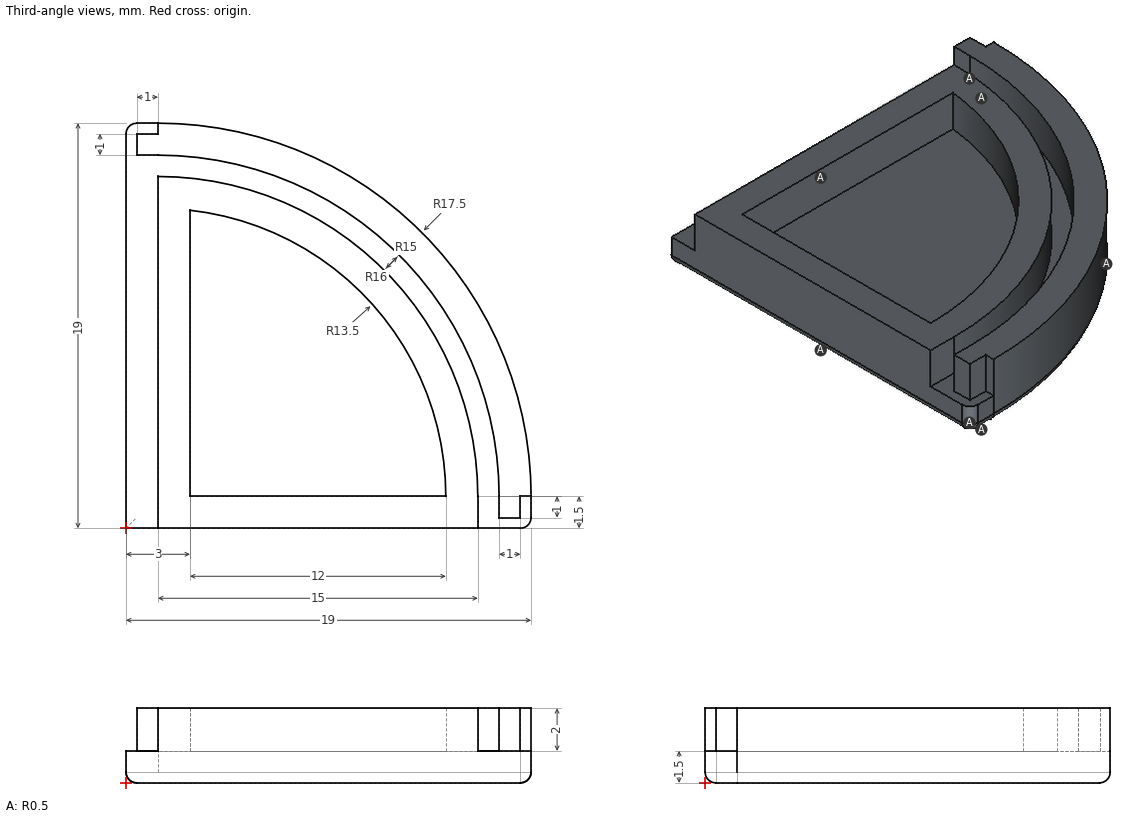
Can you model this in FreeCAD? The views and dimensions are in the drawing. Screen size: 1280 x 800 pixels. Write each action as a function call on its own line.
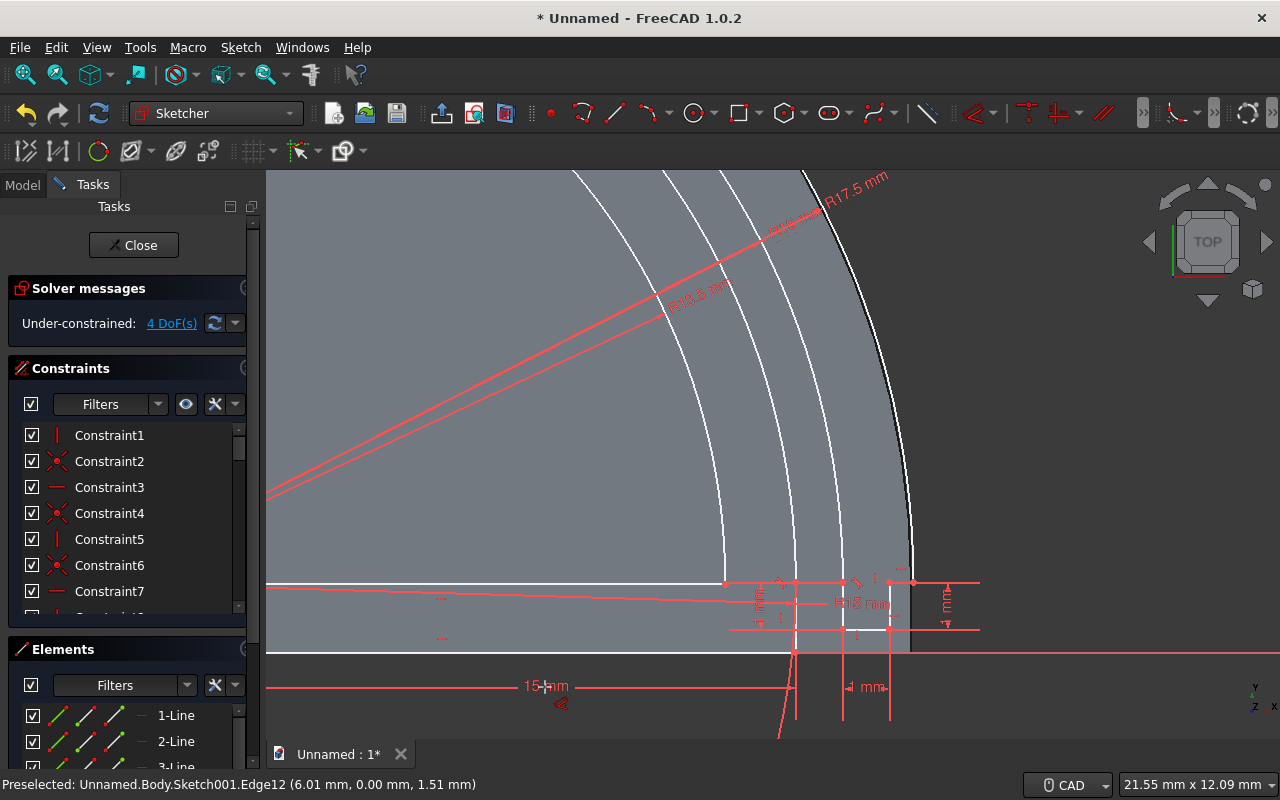
click(555, 584)
click(510, 618)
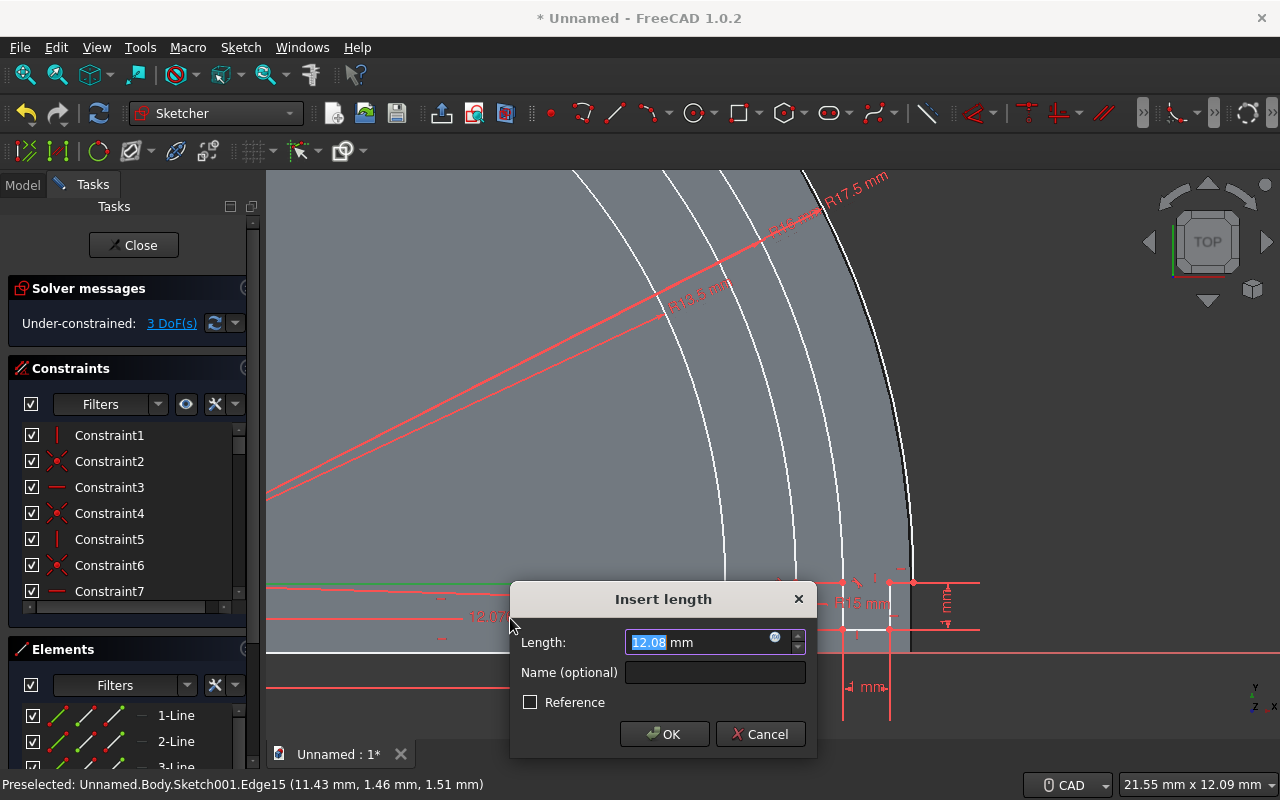
text(12)
key(Return)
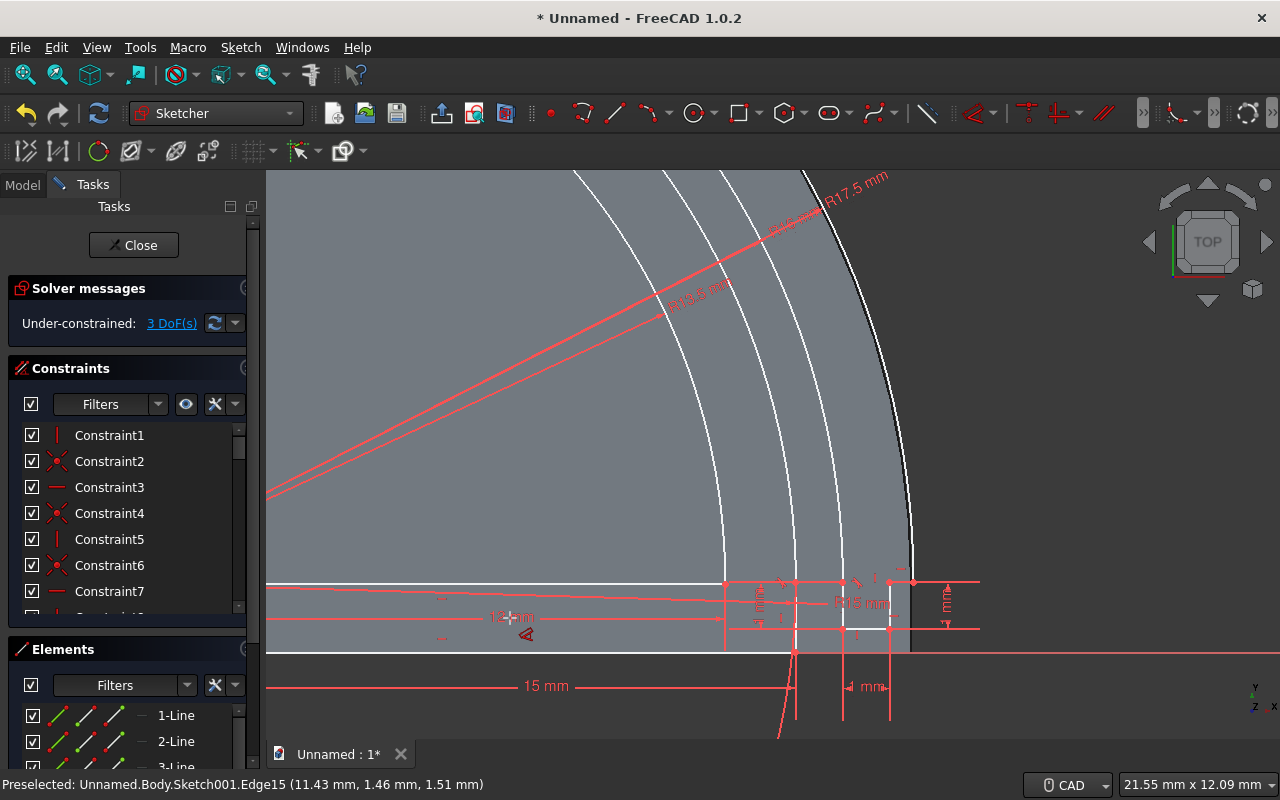
scroll(844, 599, down, 5)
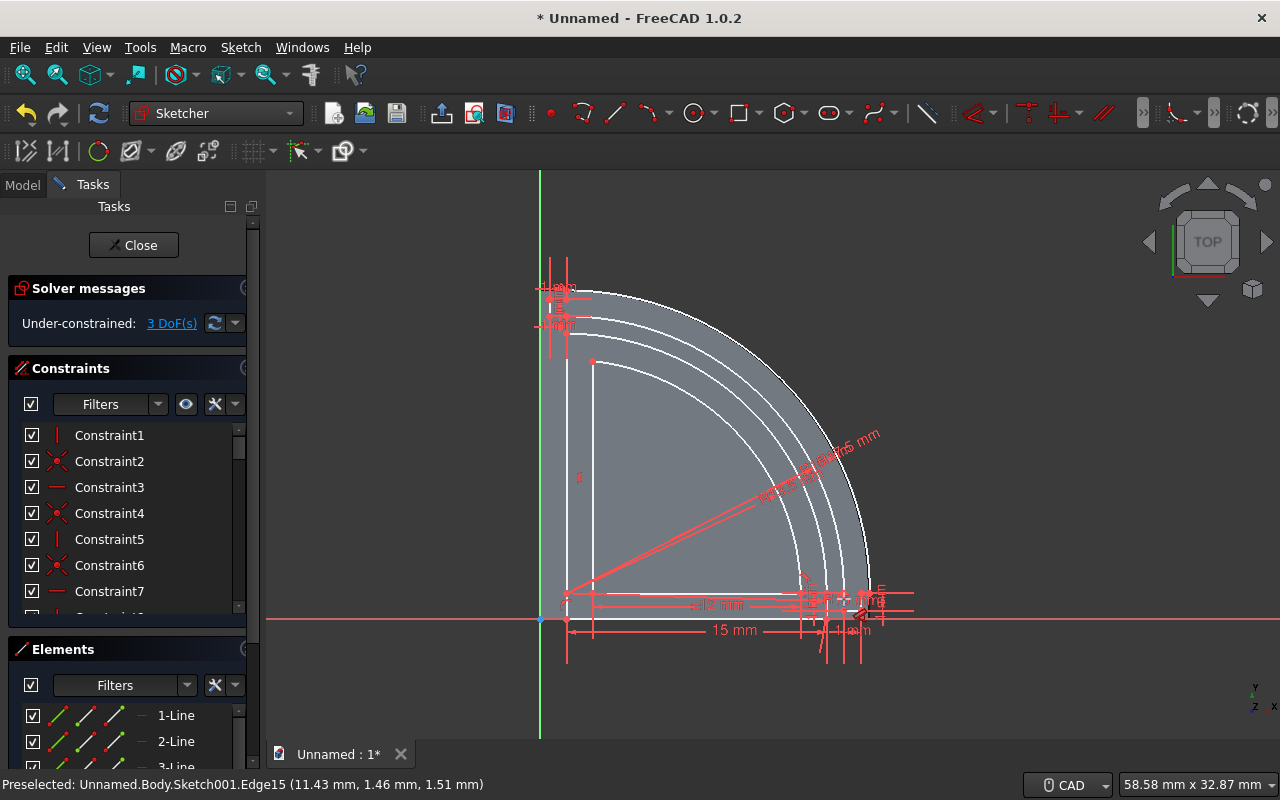
click(593, 594)
click(567, 653)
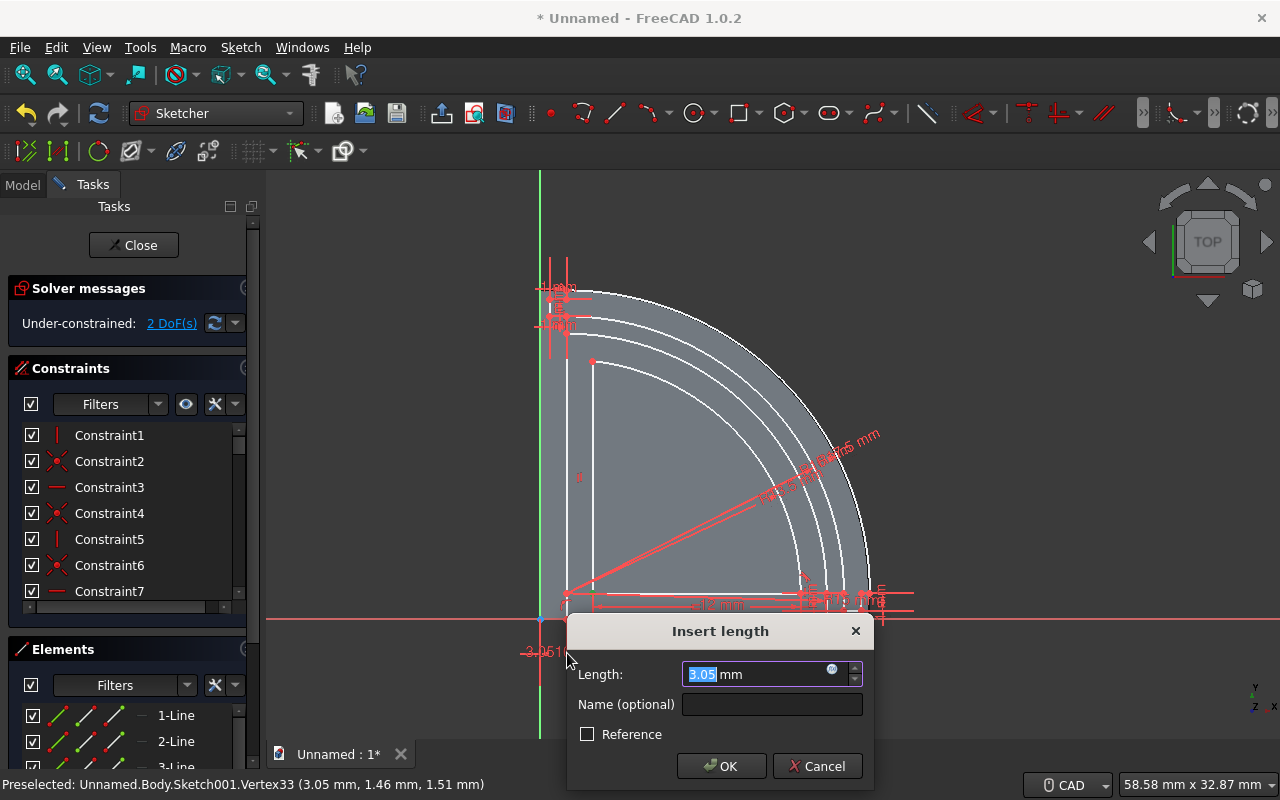
text(3)
key(Return)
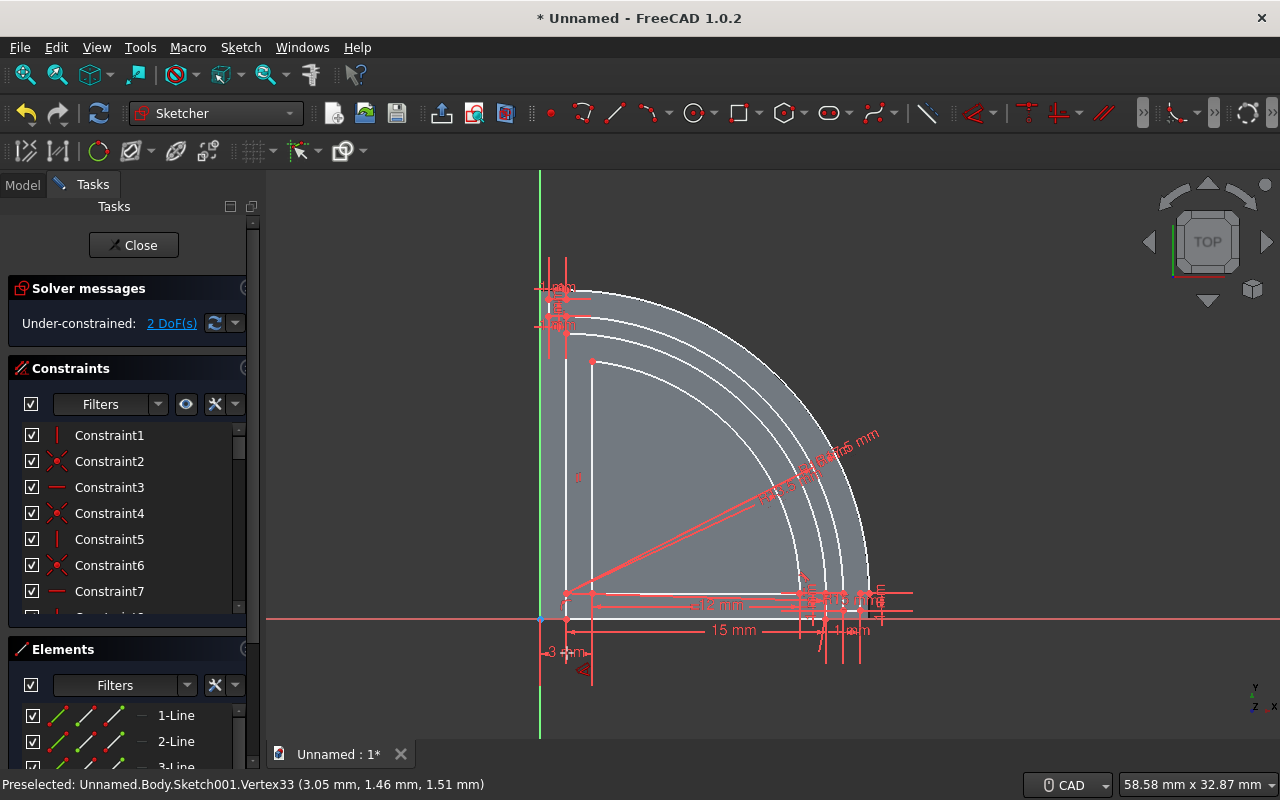
scroll(826, 609, up, 3)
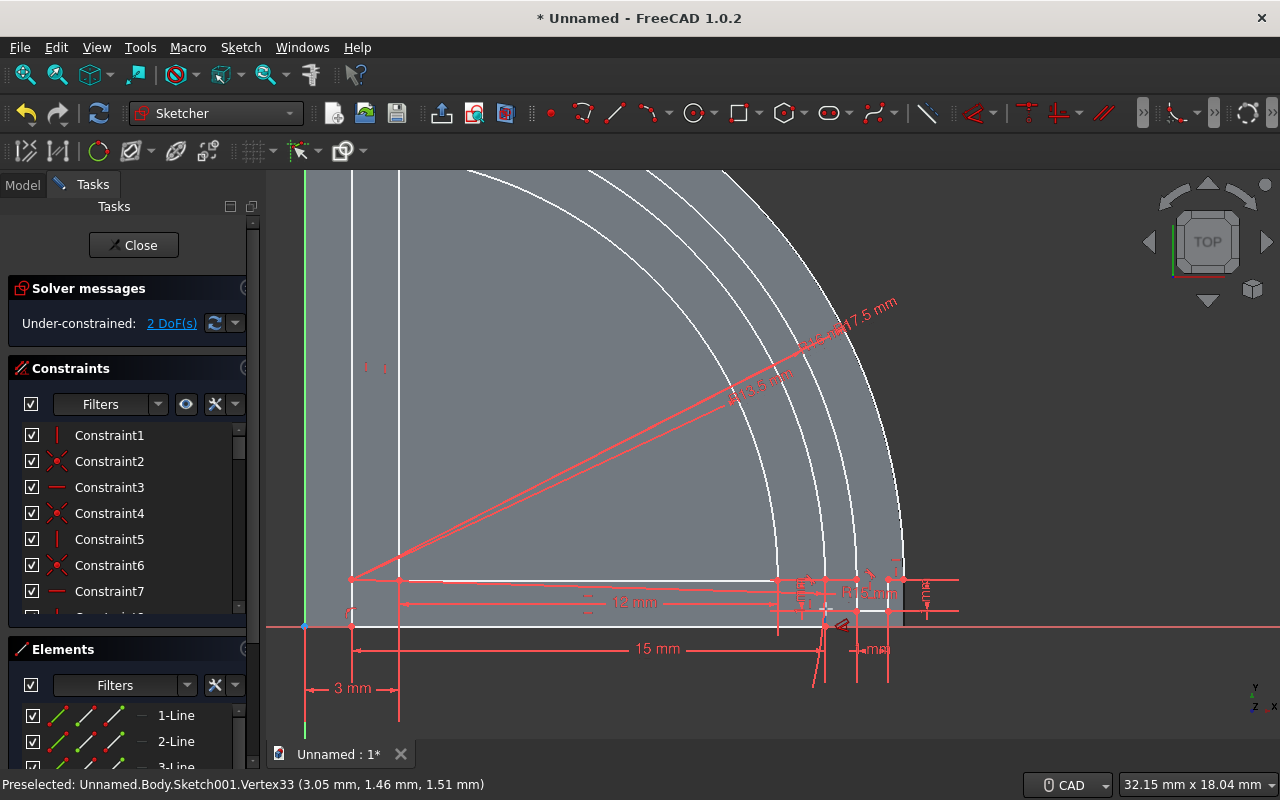
click(825, 608)
click(719, 603)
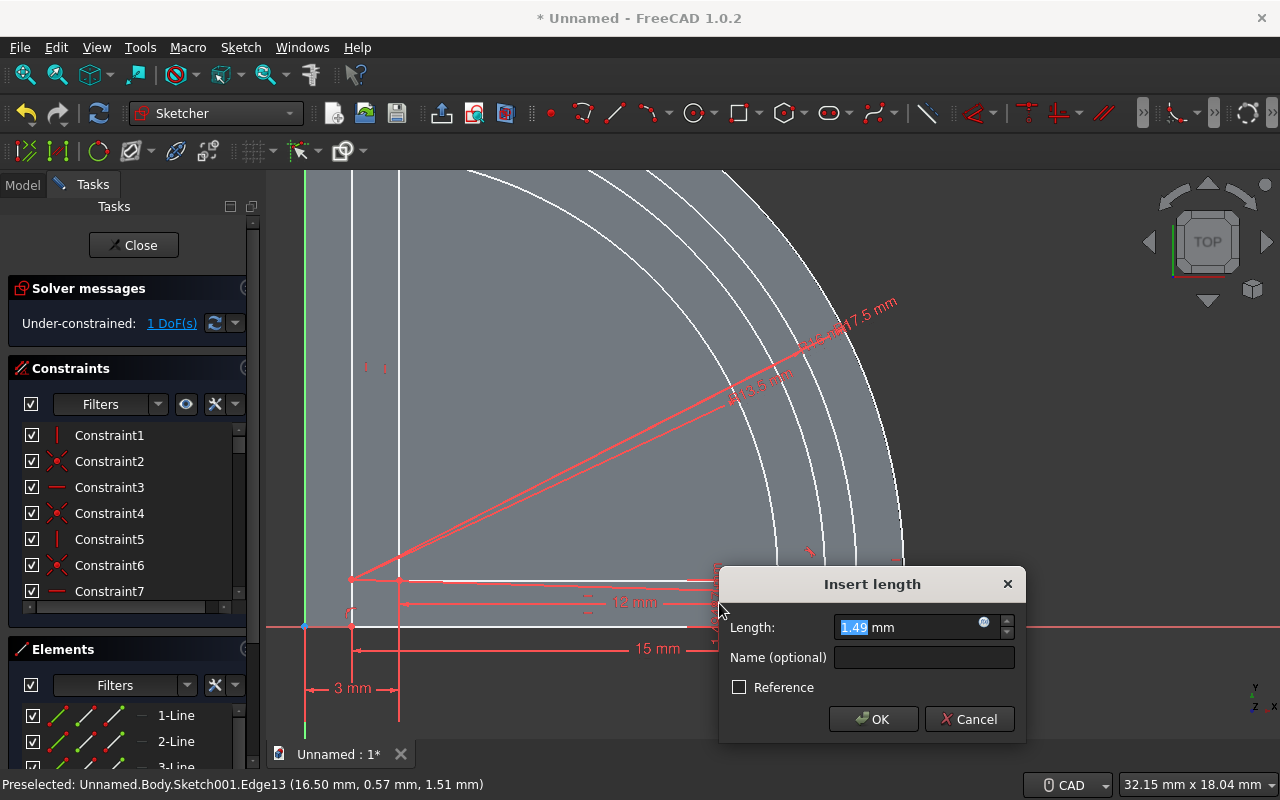
text(1.5)
key(Return)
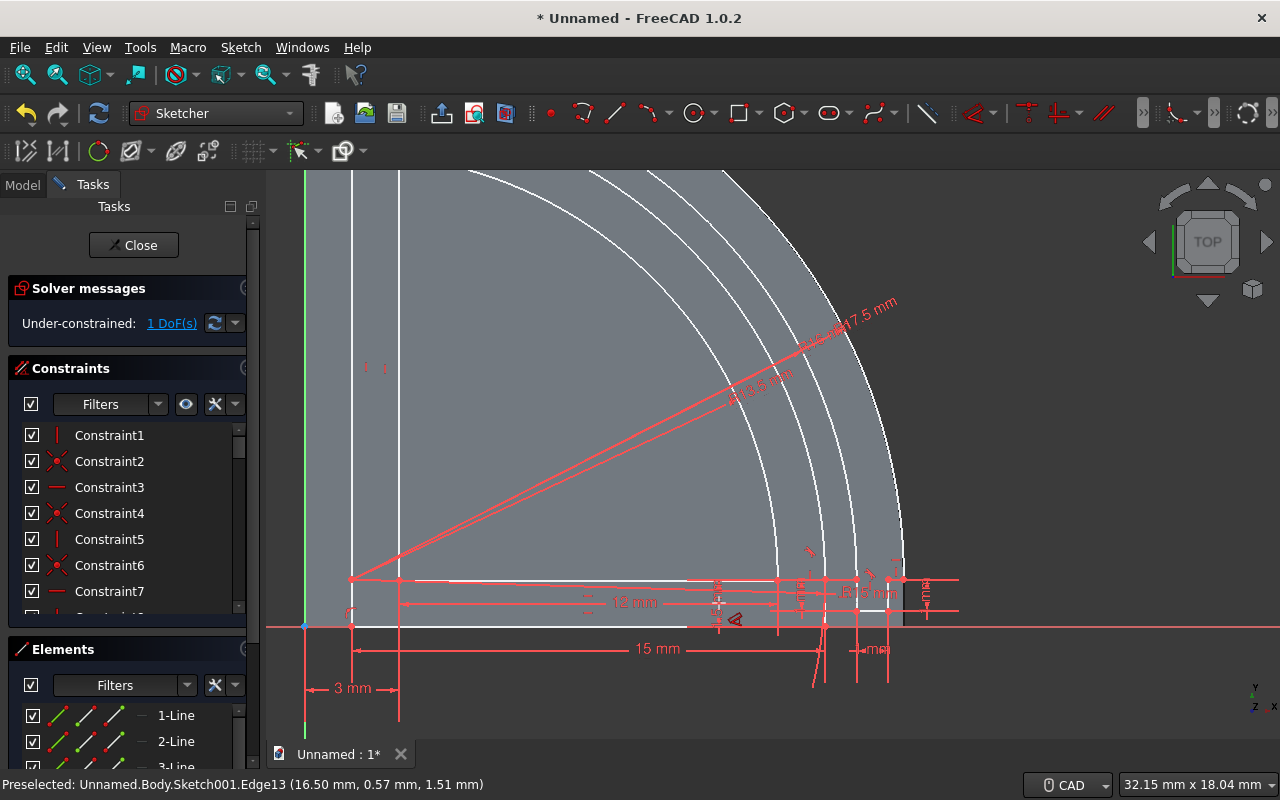
click(778, 581)
click(812, 615)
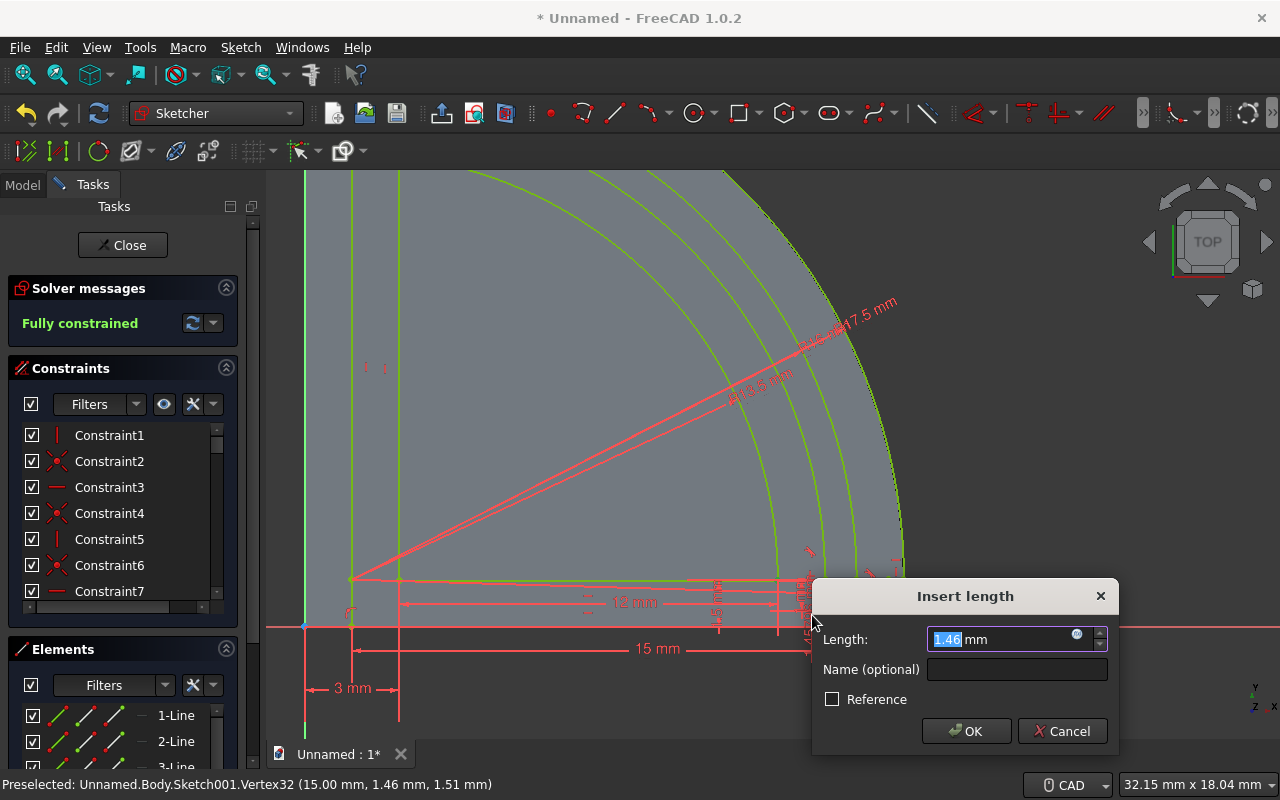
text(1.5)
key(Return)
key(Escape)